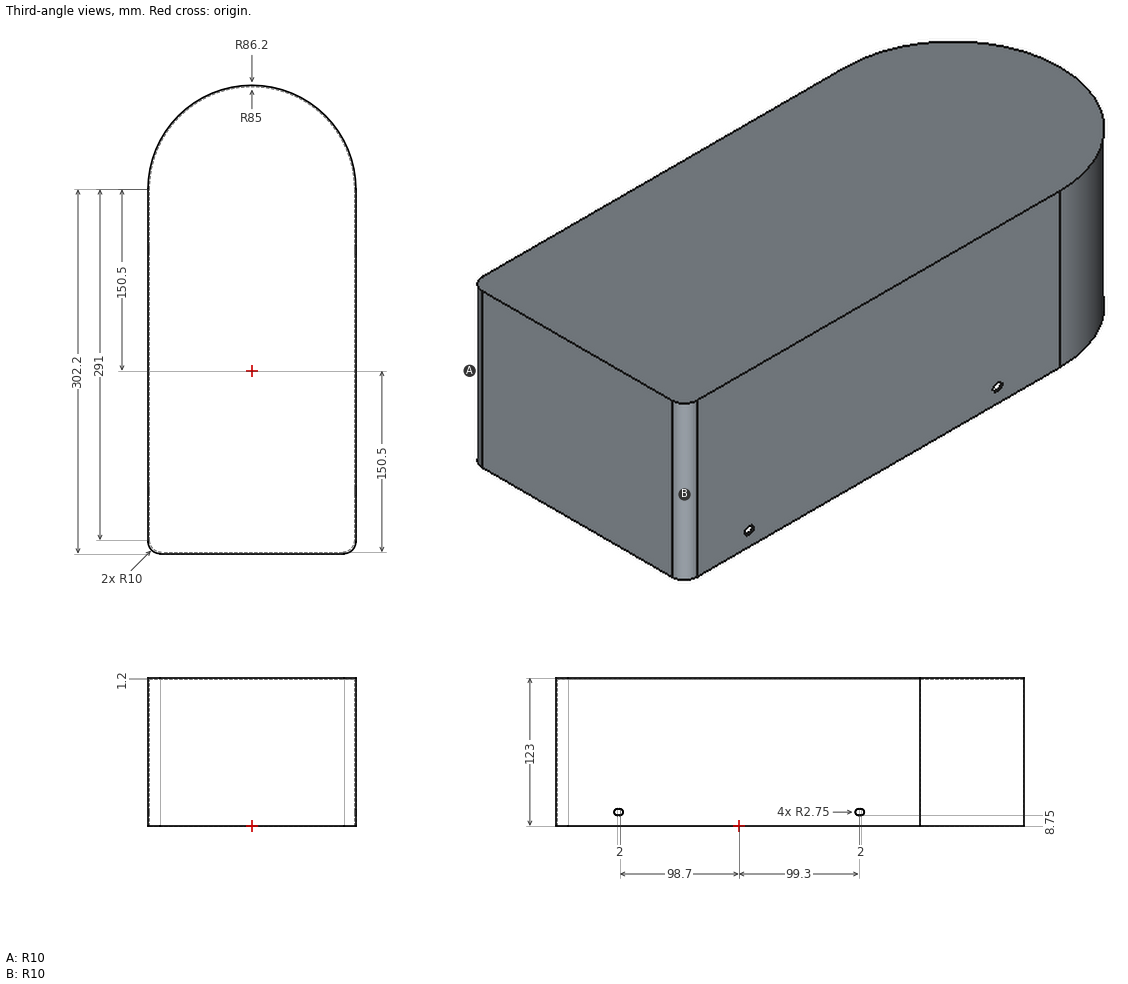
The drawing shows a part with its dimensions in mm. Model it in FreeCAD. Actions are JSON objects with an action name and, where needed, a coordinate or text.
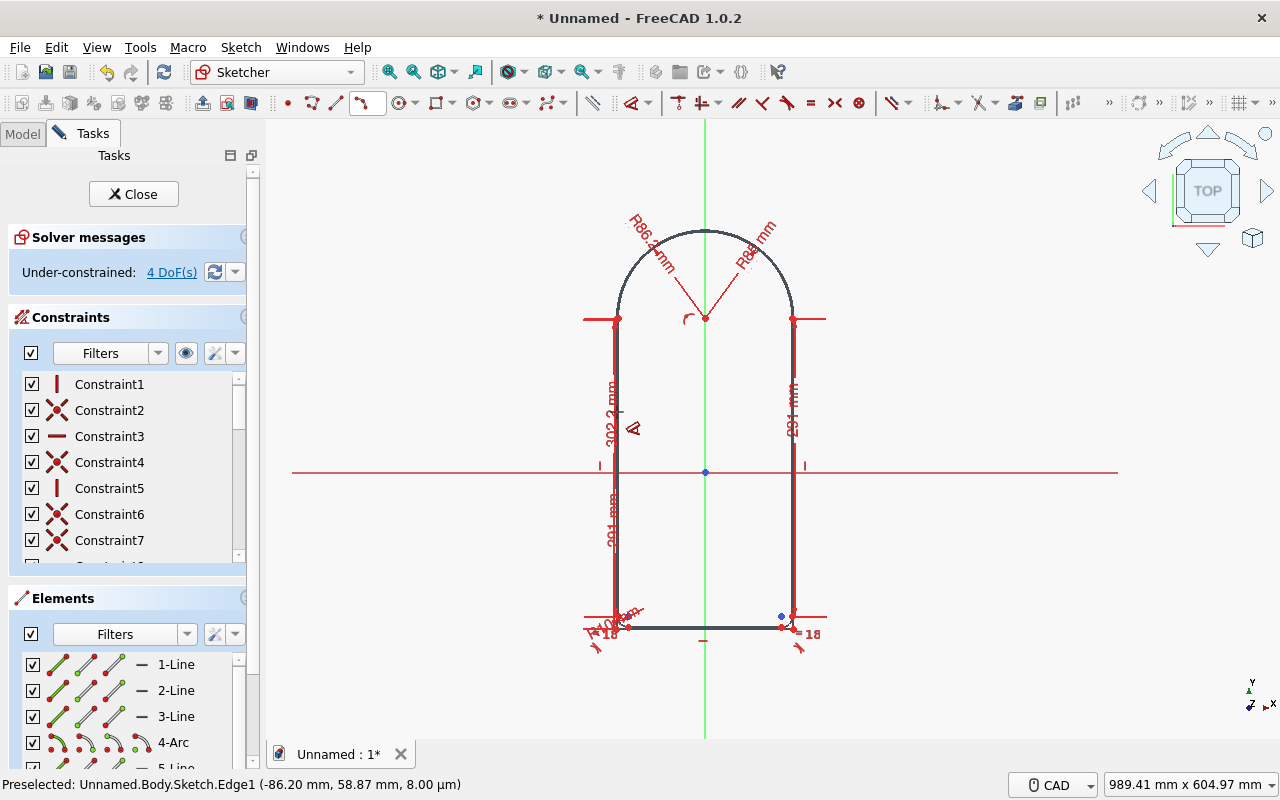
{"action": "scroll", "coordinate": [793, 536], "scroll_direction": "up", "scroll_amount": 13}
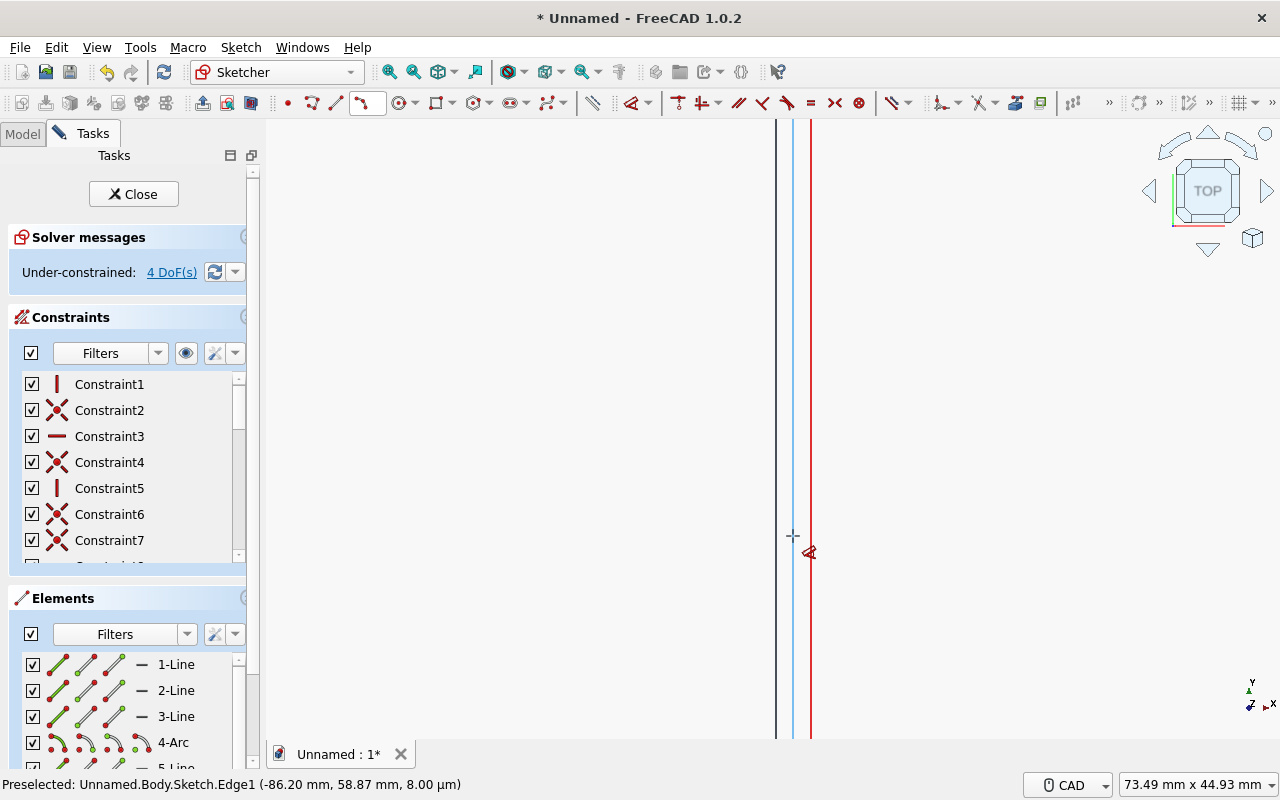
{"action": "left_click", "coordinate": [793, 533]}
{"action": "left_click", "coordinate": [827, 429]}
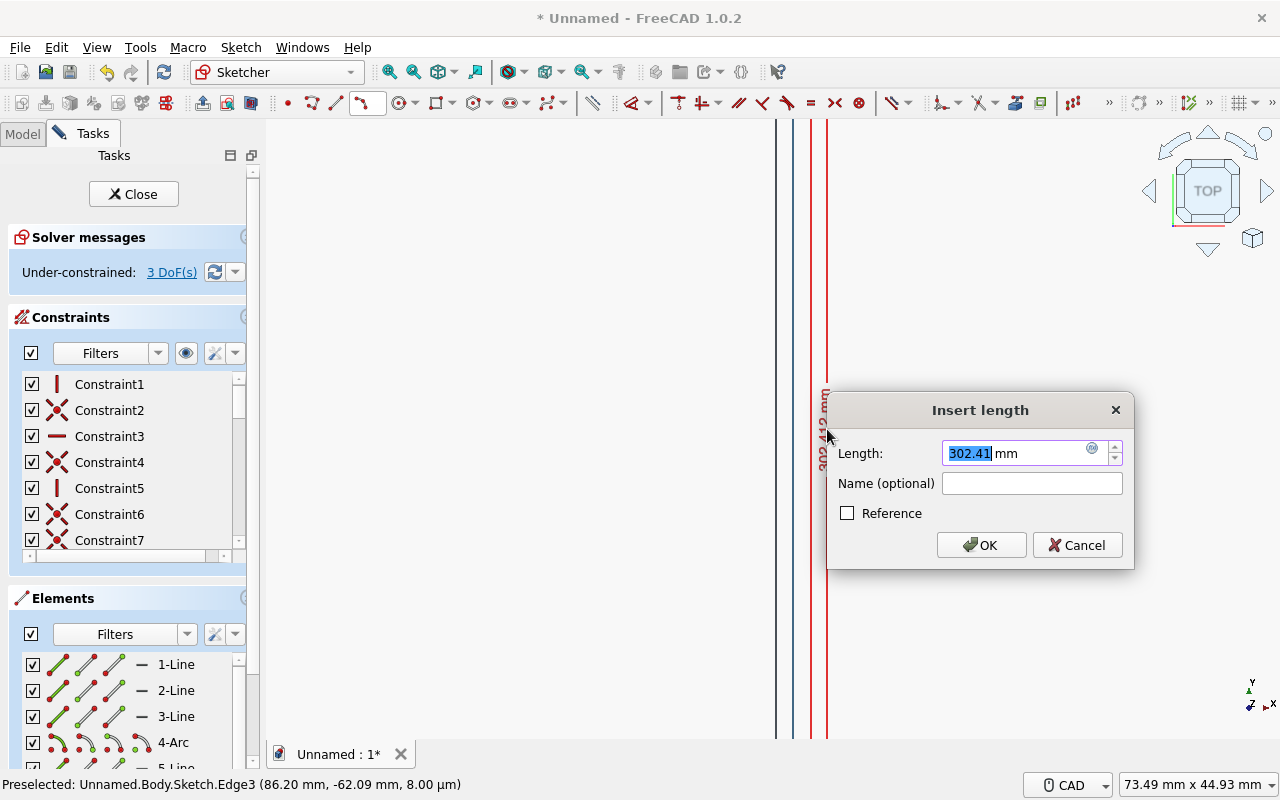
{"action": "type", "text": "302.2"}
{"action": "key", "text": "Return"}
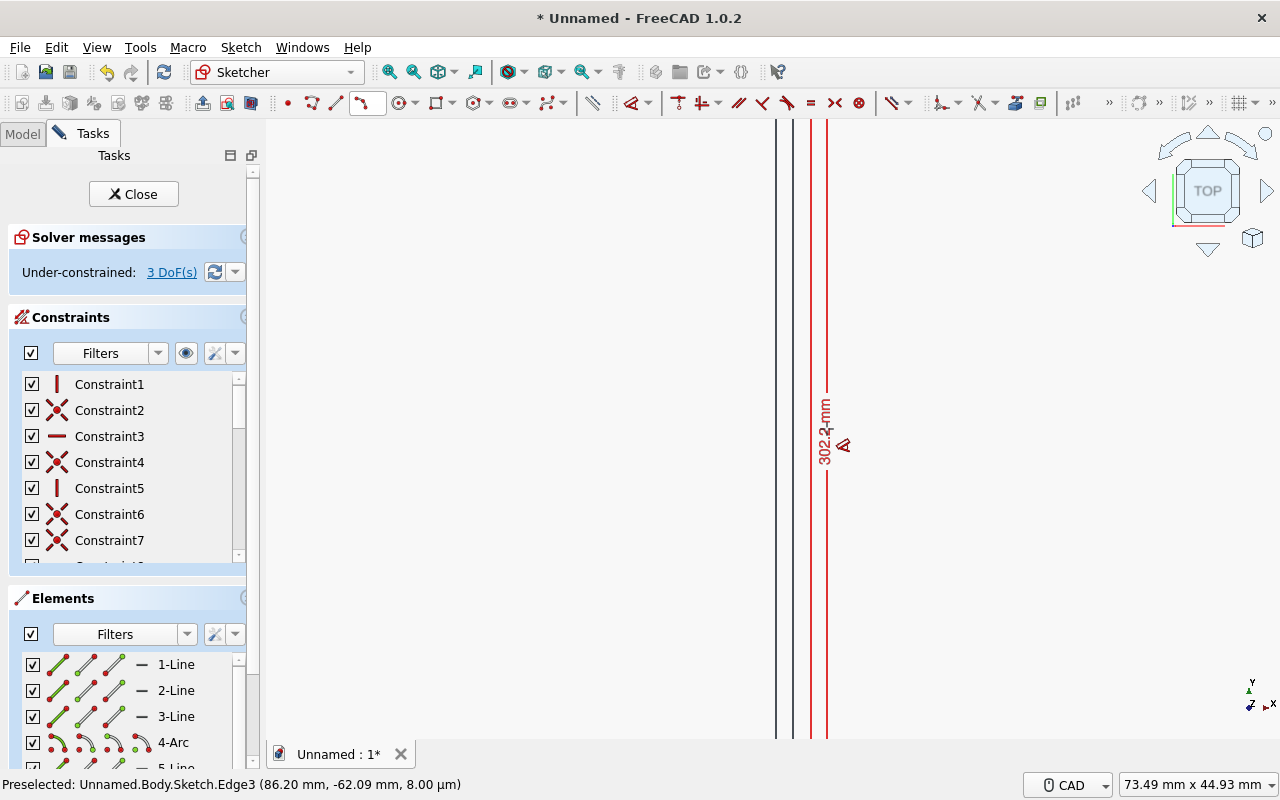
{"action": "scroll", "coordinate": [793, 536], "scroll_direction": "down", "scroll_amount": 13}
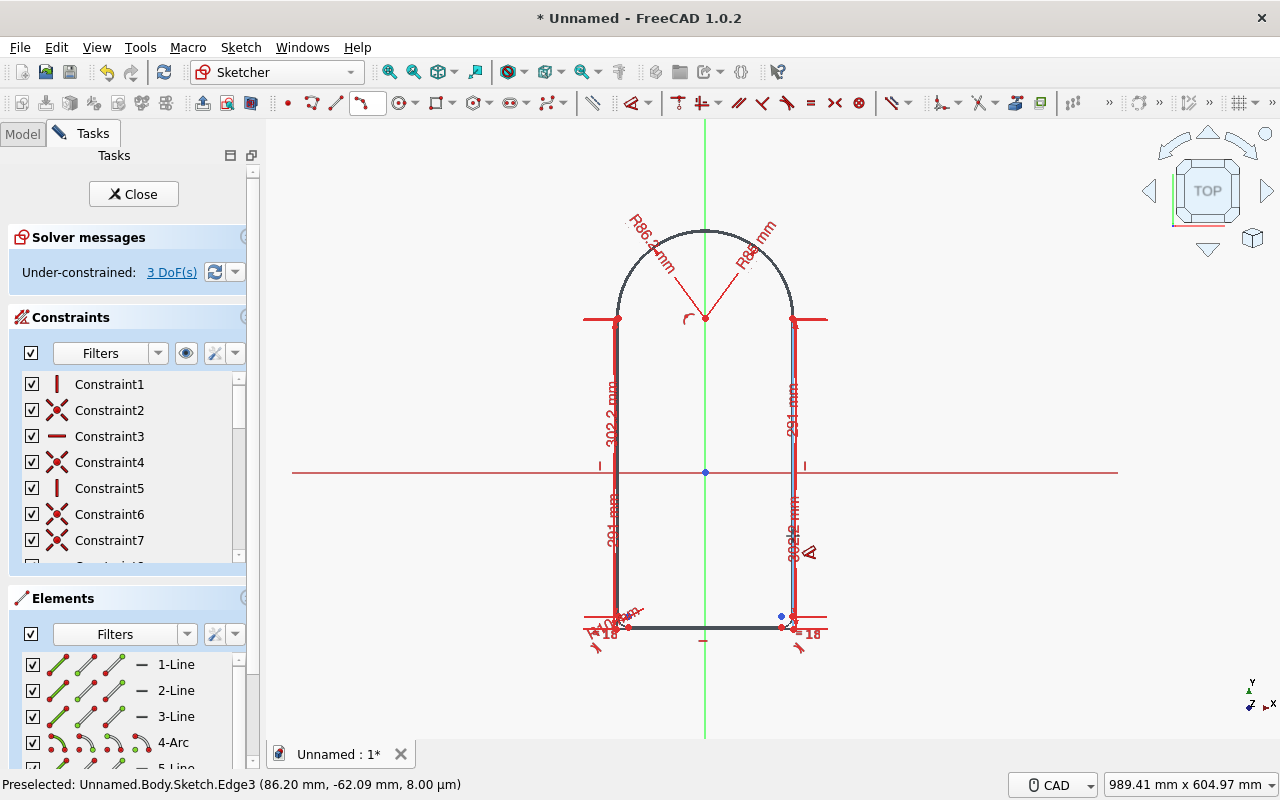
{"action": "scroll", "coordinate": [617, 320], "scroll_direction": "up", "scroll_amount": 11}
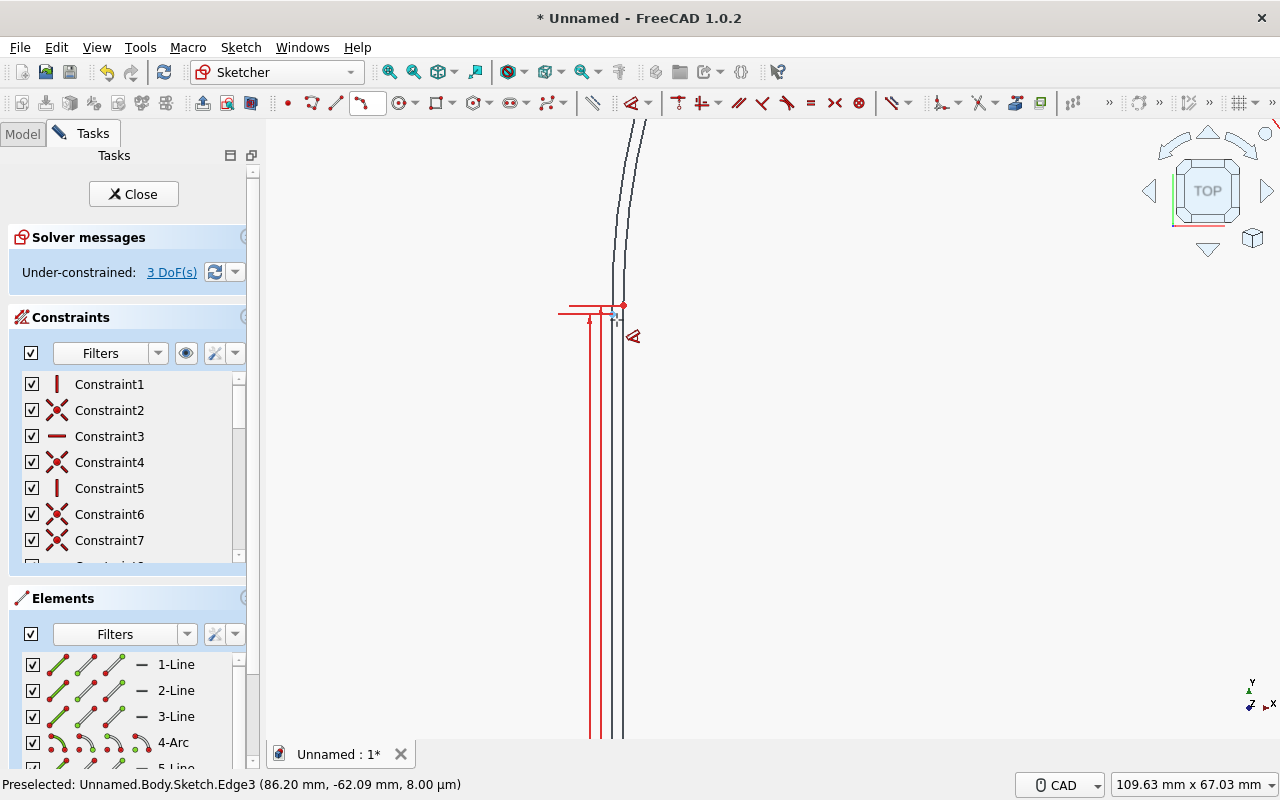
{"action": "left_click", "coordinate": [612, 314]}
{"action": "left_click", "coordinate": [578, 513]}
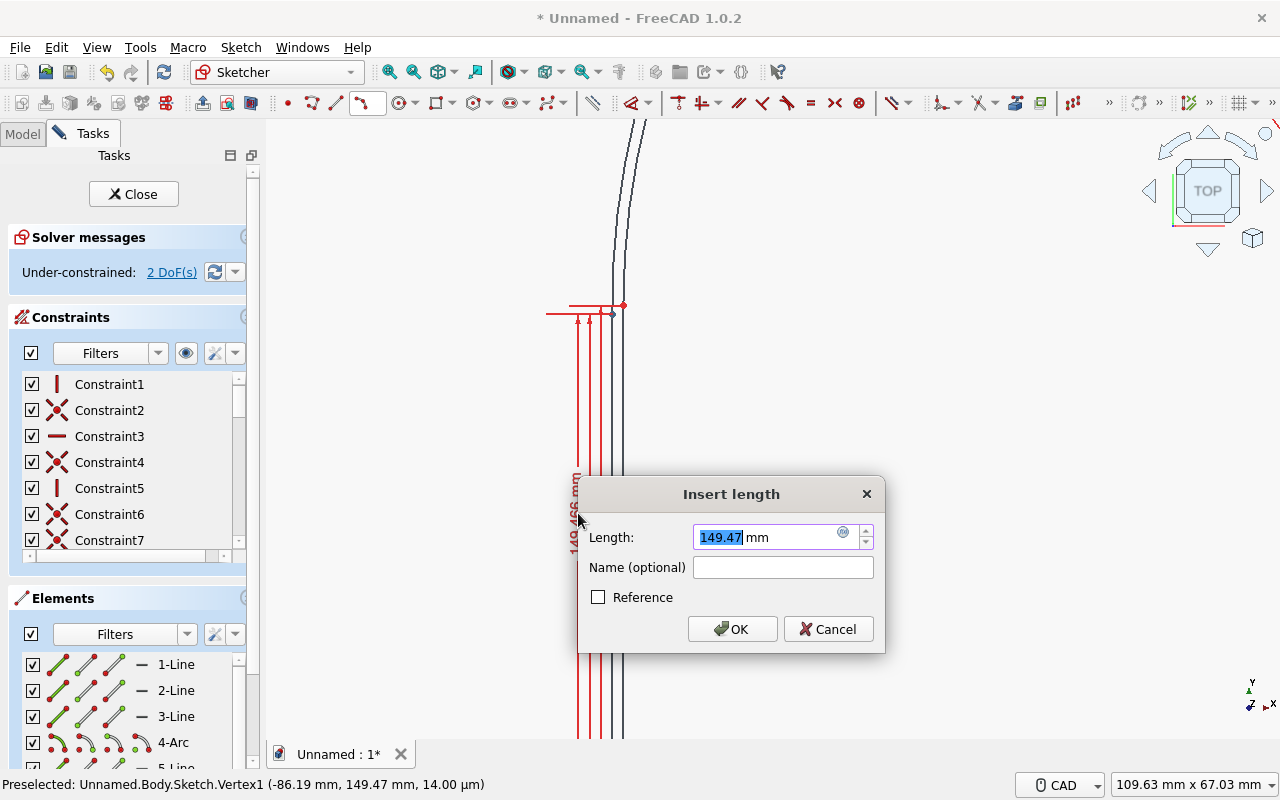
{"action": "type", "text": "150.5"}
{"action": "key", "text": "Return"}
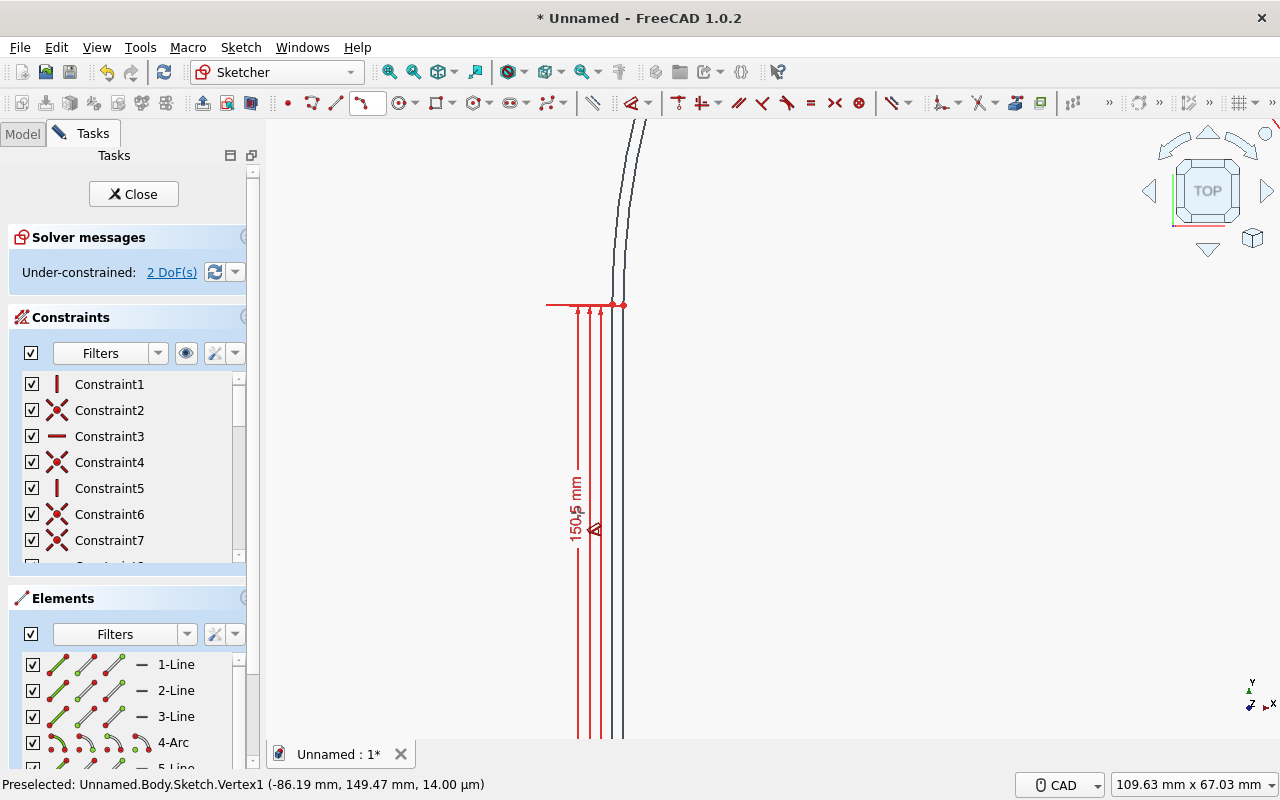
{"action": "scroll", "coordinate": [617, 320], "scroll_direction": "down", "scroll_amount": 11}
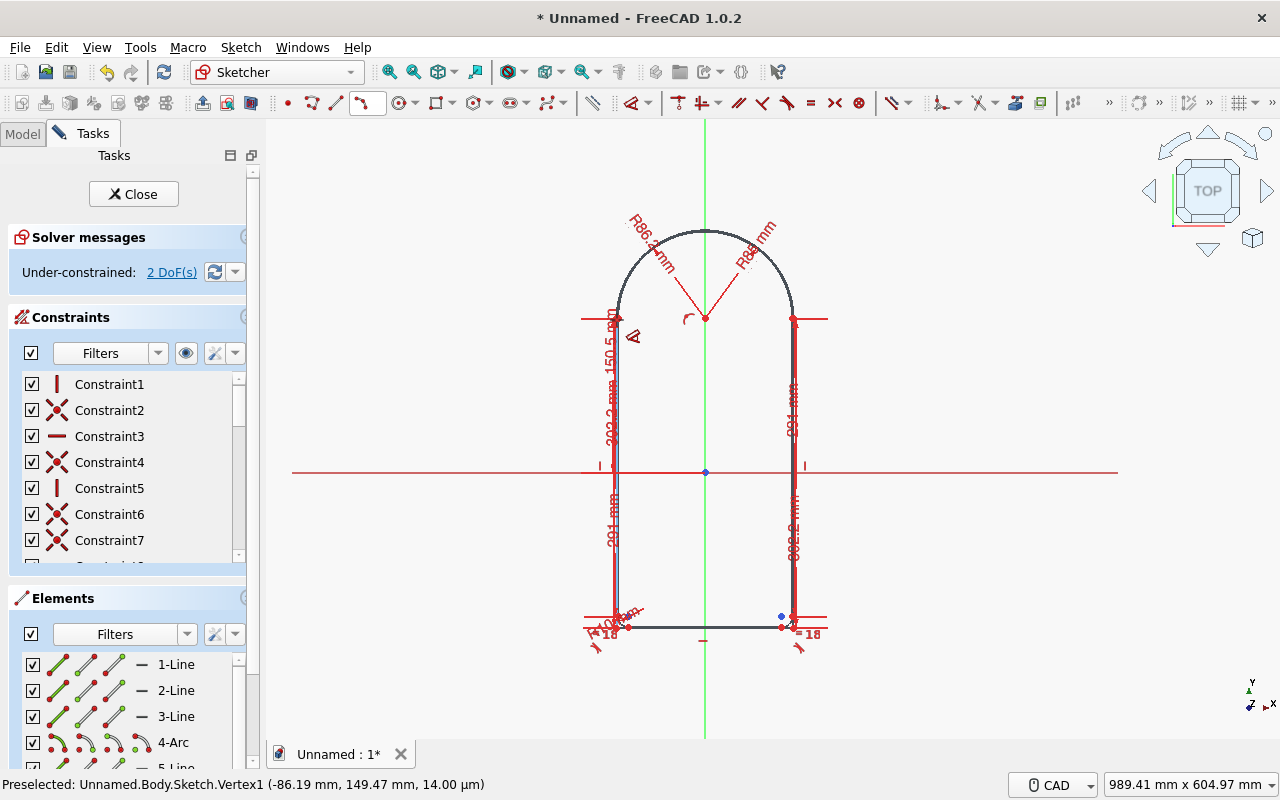
{"action": "left_click", "coordinate": [782, 627]}
{"action": "left_click", "coordinate": [816, 550]}